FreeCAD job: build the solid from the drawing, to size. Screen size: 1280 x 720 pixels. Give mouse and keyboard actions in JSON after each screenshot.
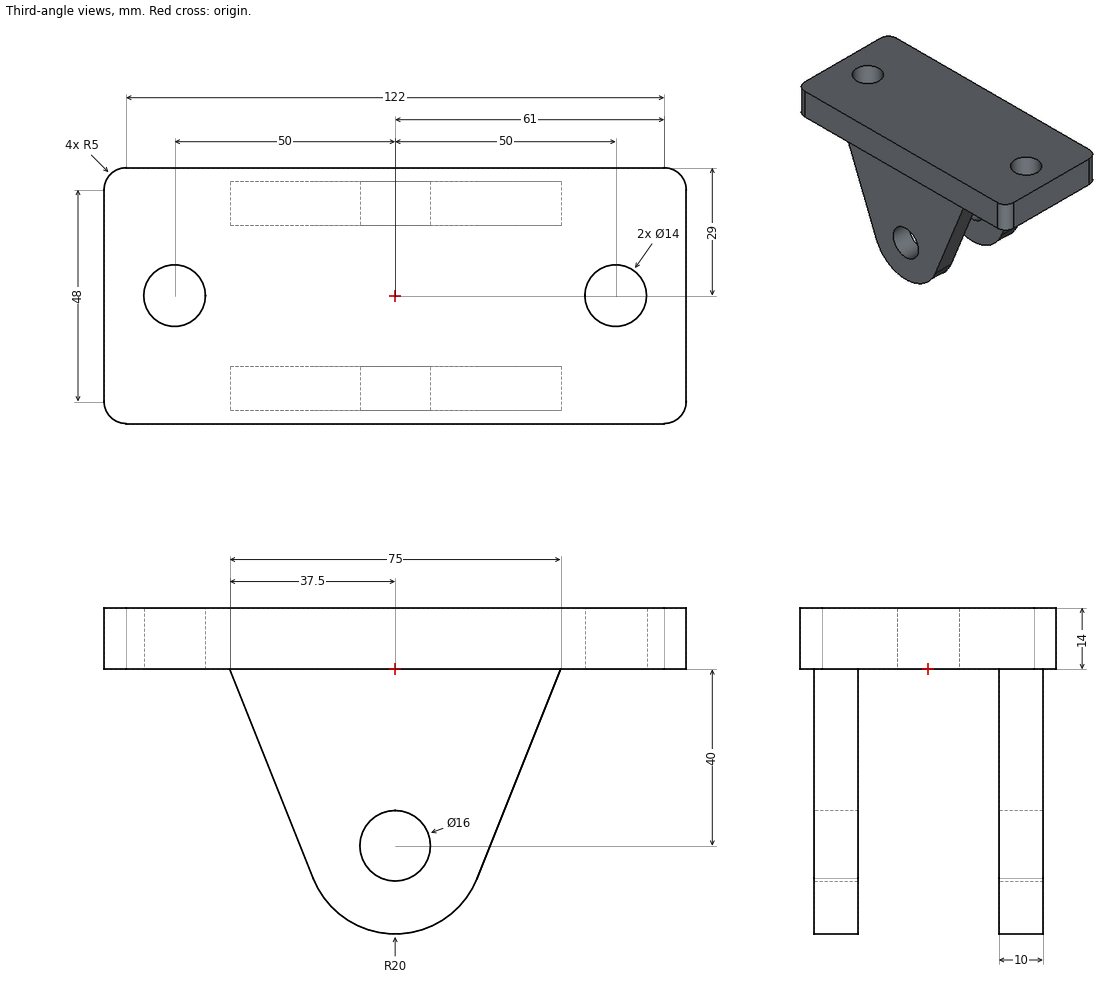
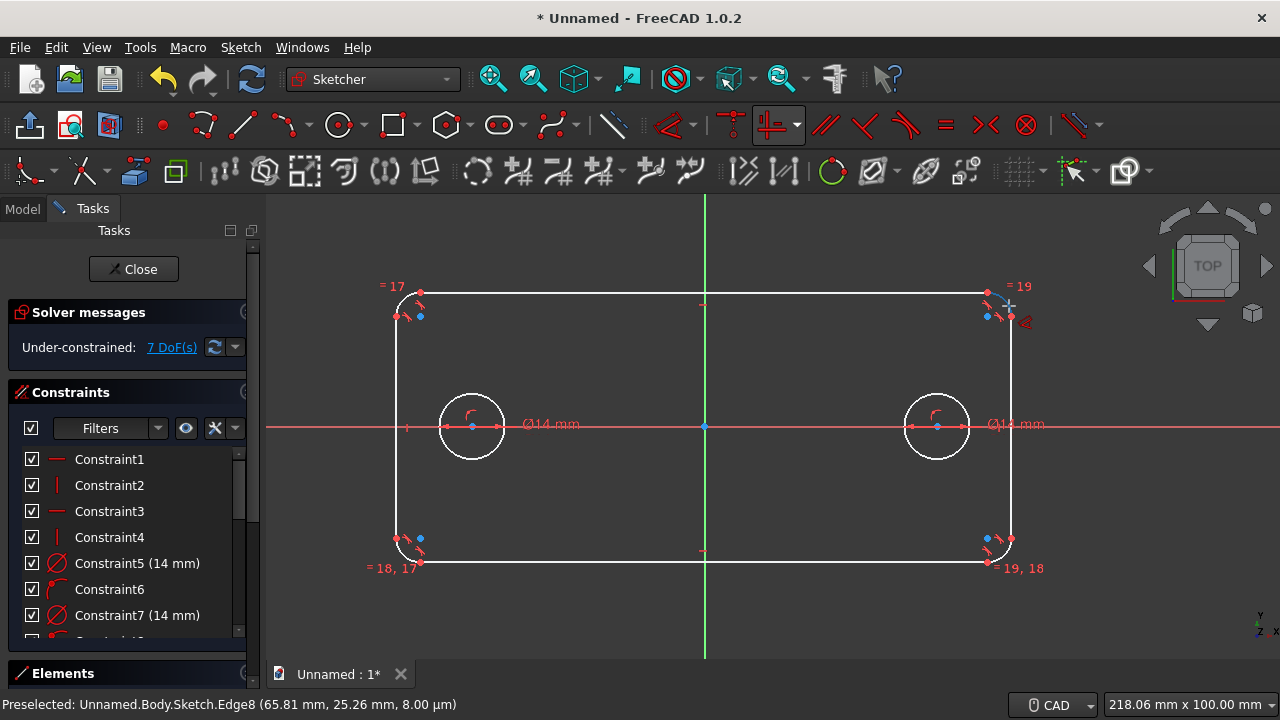
{"action": "scroll", "coordinate": [409, 295], "scroll_direction": "up", "scroll_amount": 3}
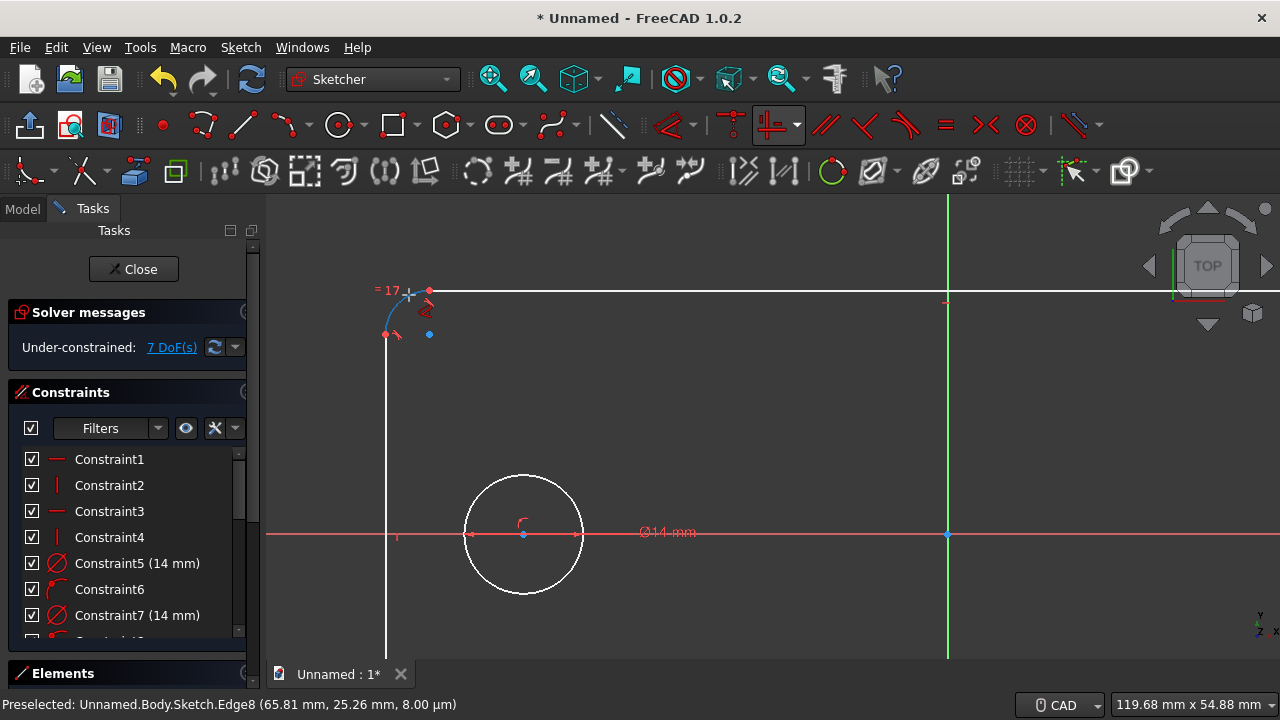
{"action": "left_click", "coordinate": [409, 296]}
{"action": "left_click", "coordinate": [394, 268]}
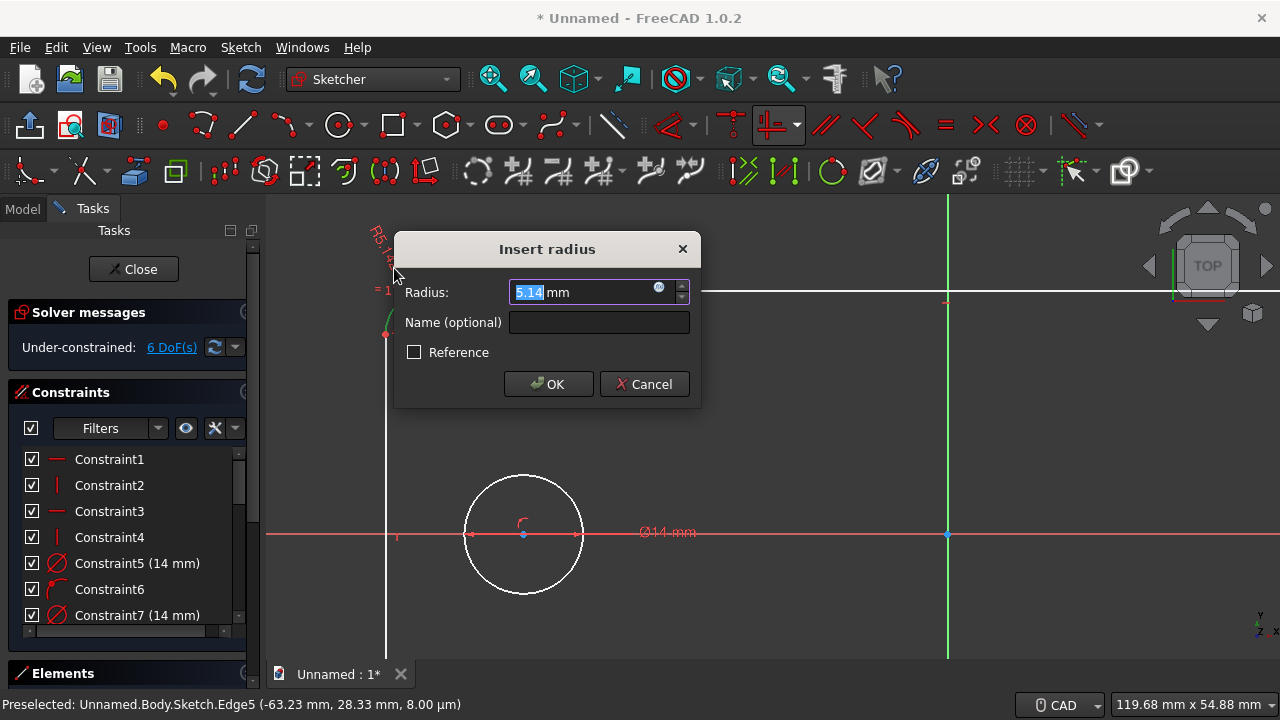
{"action": "type", "text": "5"}
{"action": "key", "text": "Return"}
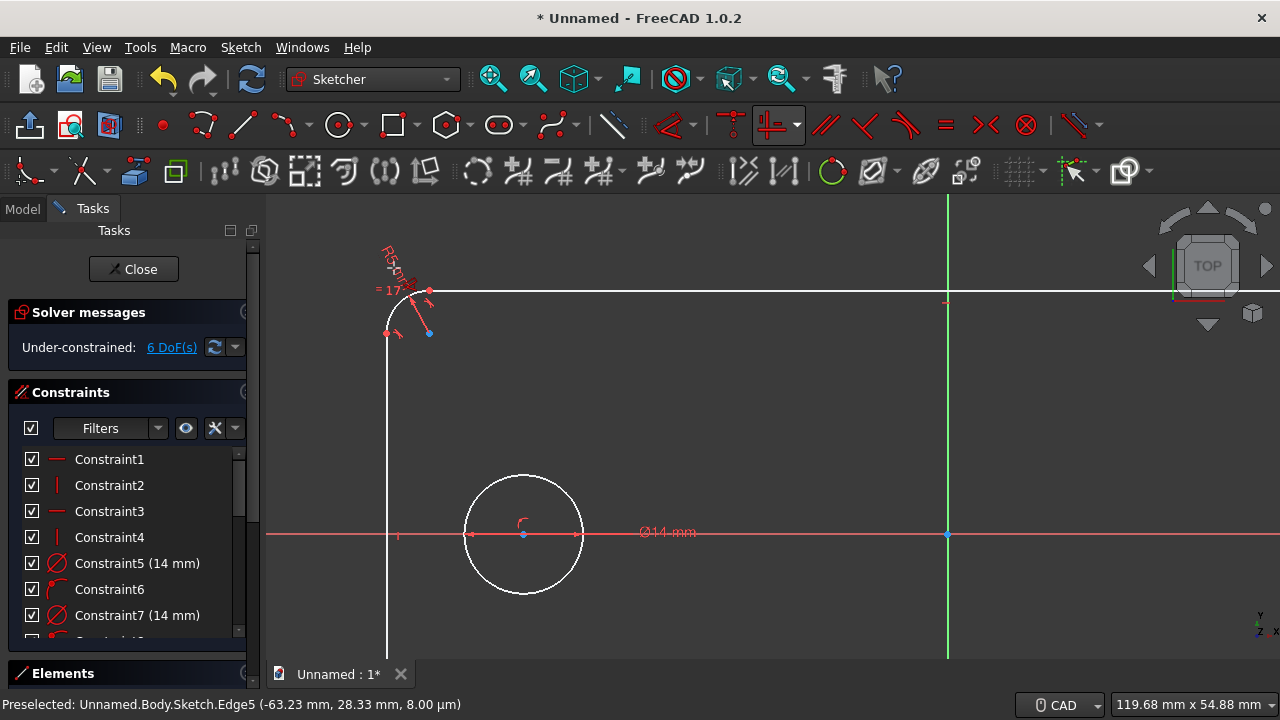
{"action": "left_click", "coordinate": [387, 455]}
{"action": "left_click", "coordinate": [353, 482]}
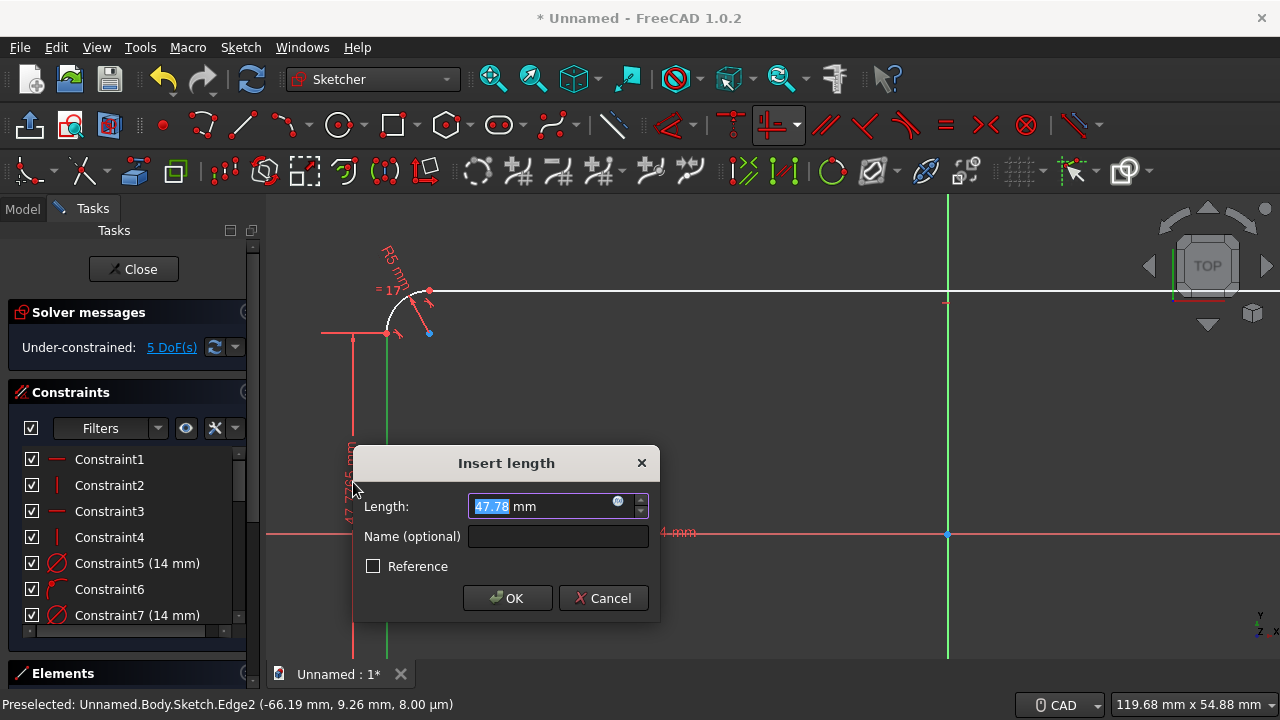
{"action": "type", "text": "48"}
{"action": "key", "text": "Return"}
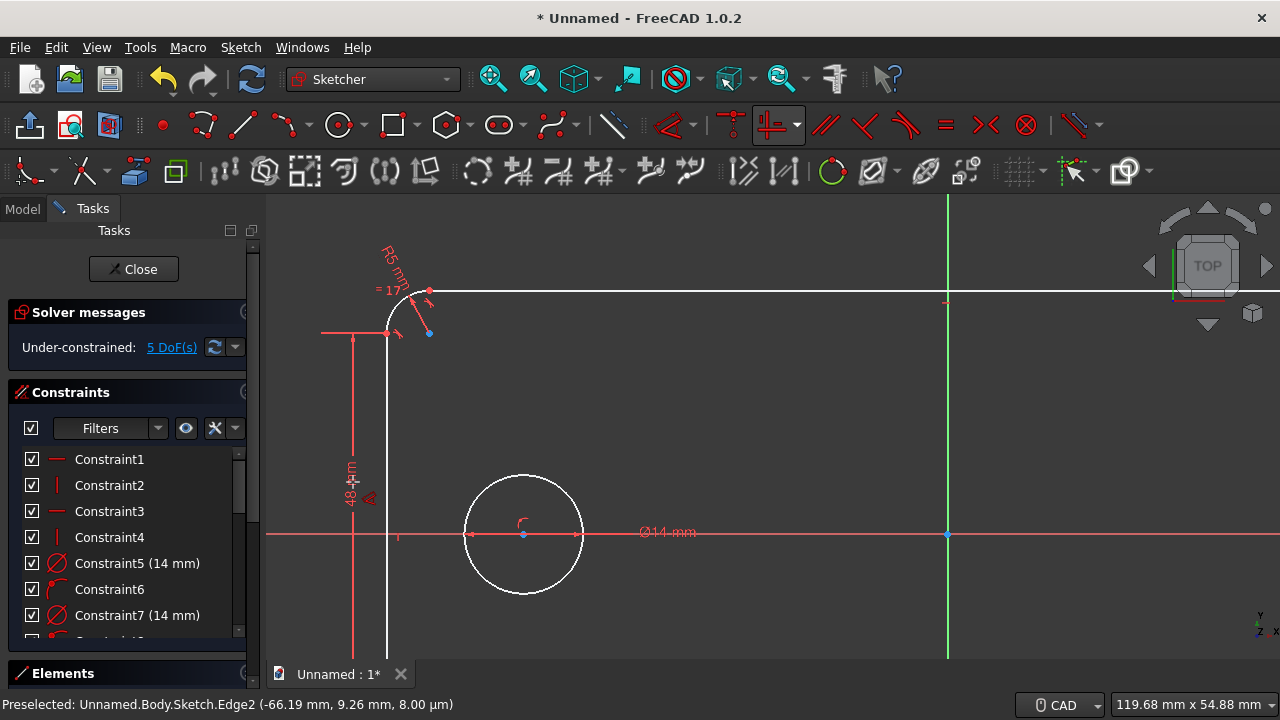
{"action": "scroll", "coordinate": [409, 295], "scroll_direction": "down", "scroll_amount": 3}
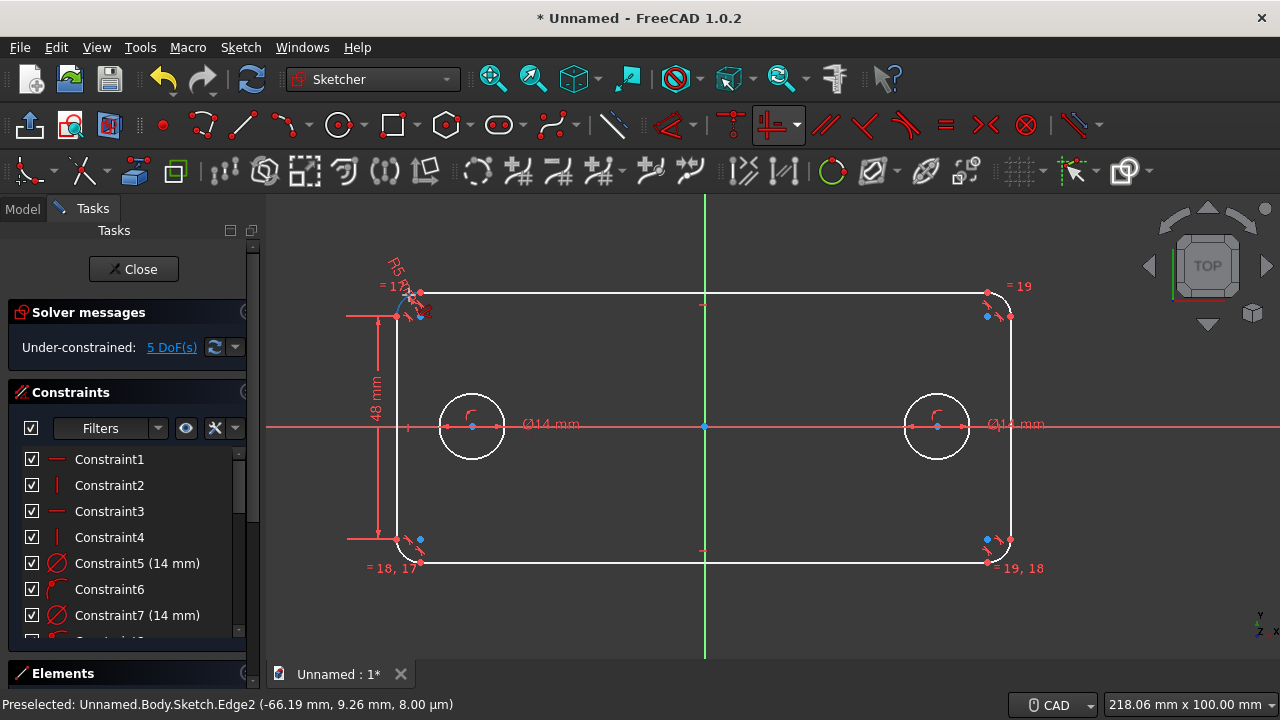
{"action": "left_click", "coordinate": [937, 426]}
{"action": "left_click", "coordinate": [821, 460]}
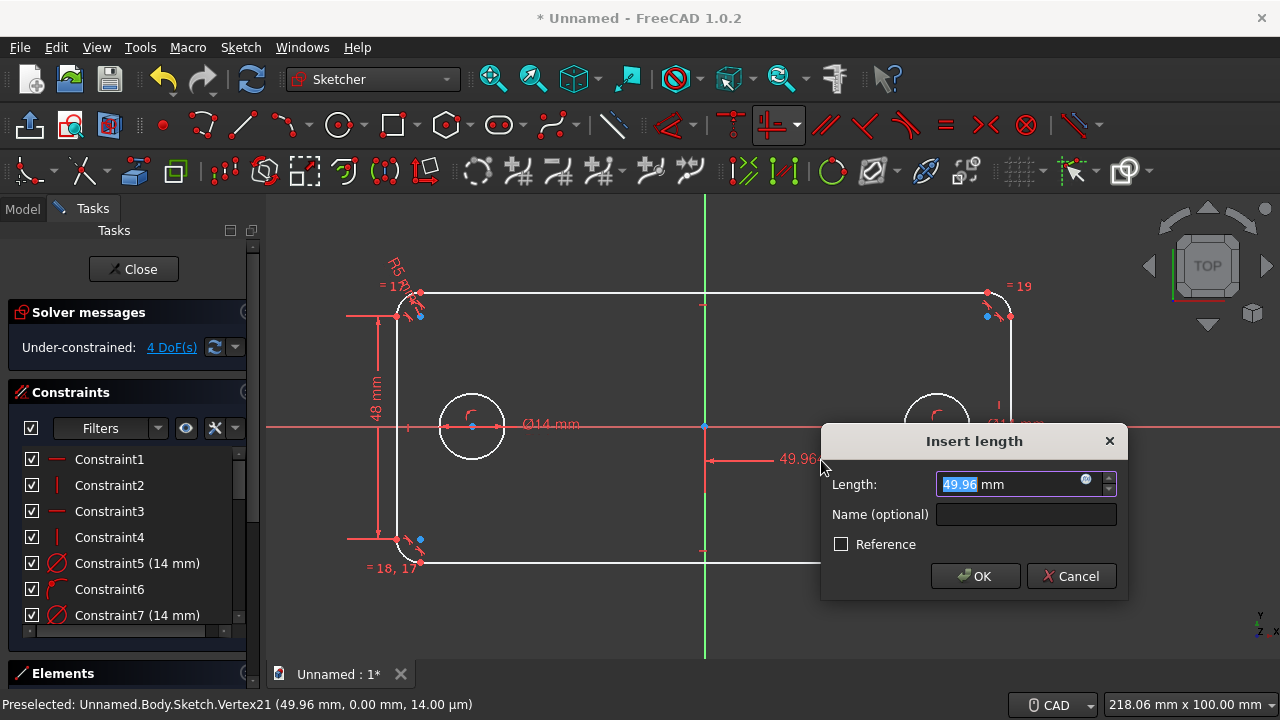
{"action": "type", "text": "50"}
{"action": "key", "text": "Return"}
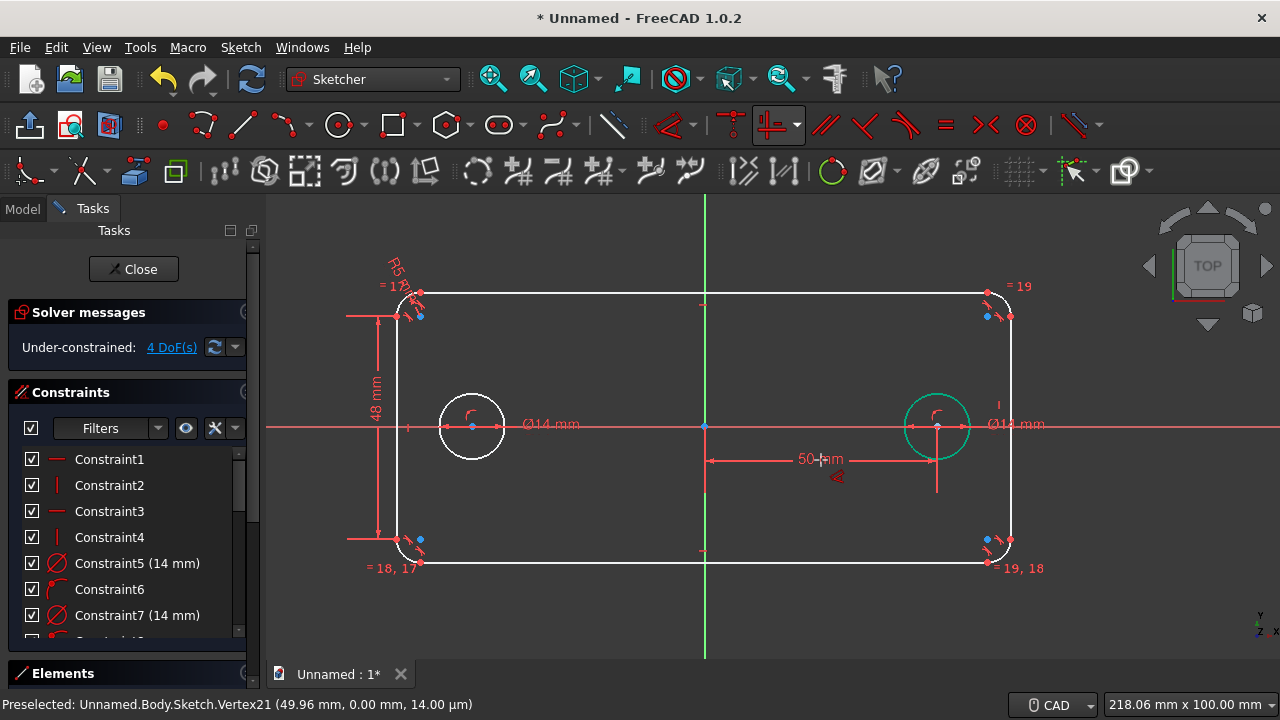
{"action": "left_click", "coordinate": [472, 426]}
{"action": "left_click", "coordinate": [588, 460]}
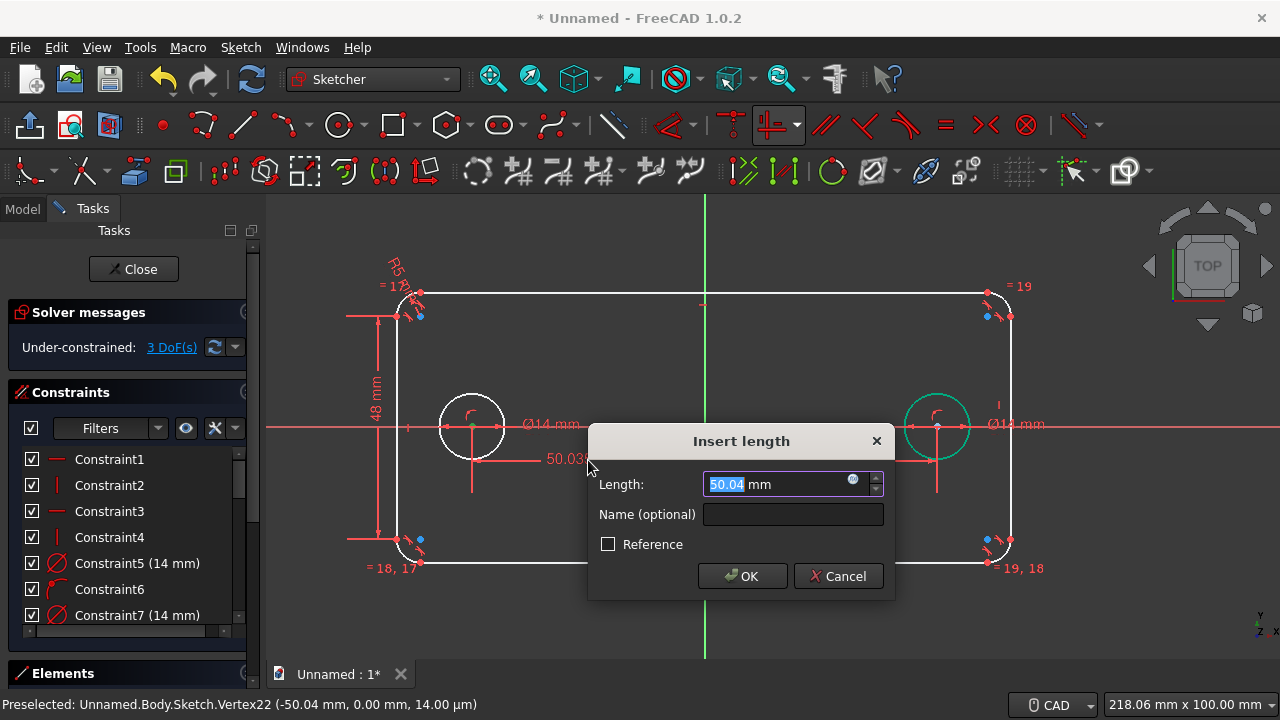
{"action": "type", "text": "50"}
{"action": "key", "text": "Return"}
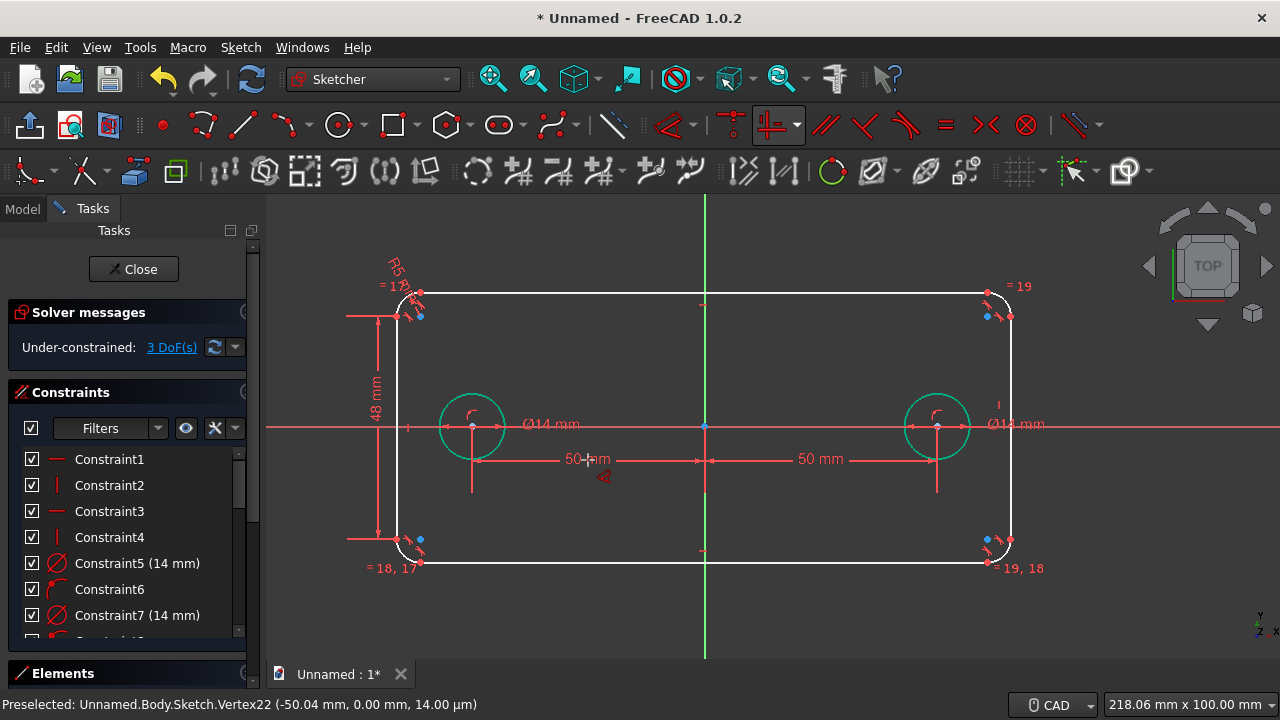
{"action": "left_click", "coordinate": [817, 293]}
{"action": "left_click", "coordinate": [573, 259]}